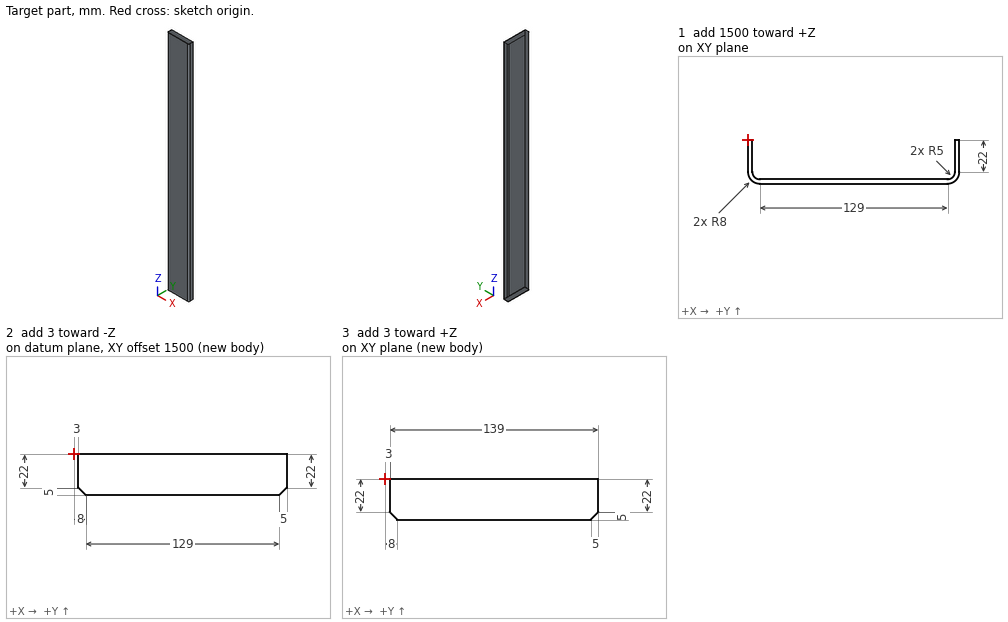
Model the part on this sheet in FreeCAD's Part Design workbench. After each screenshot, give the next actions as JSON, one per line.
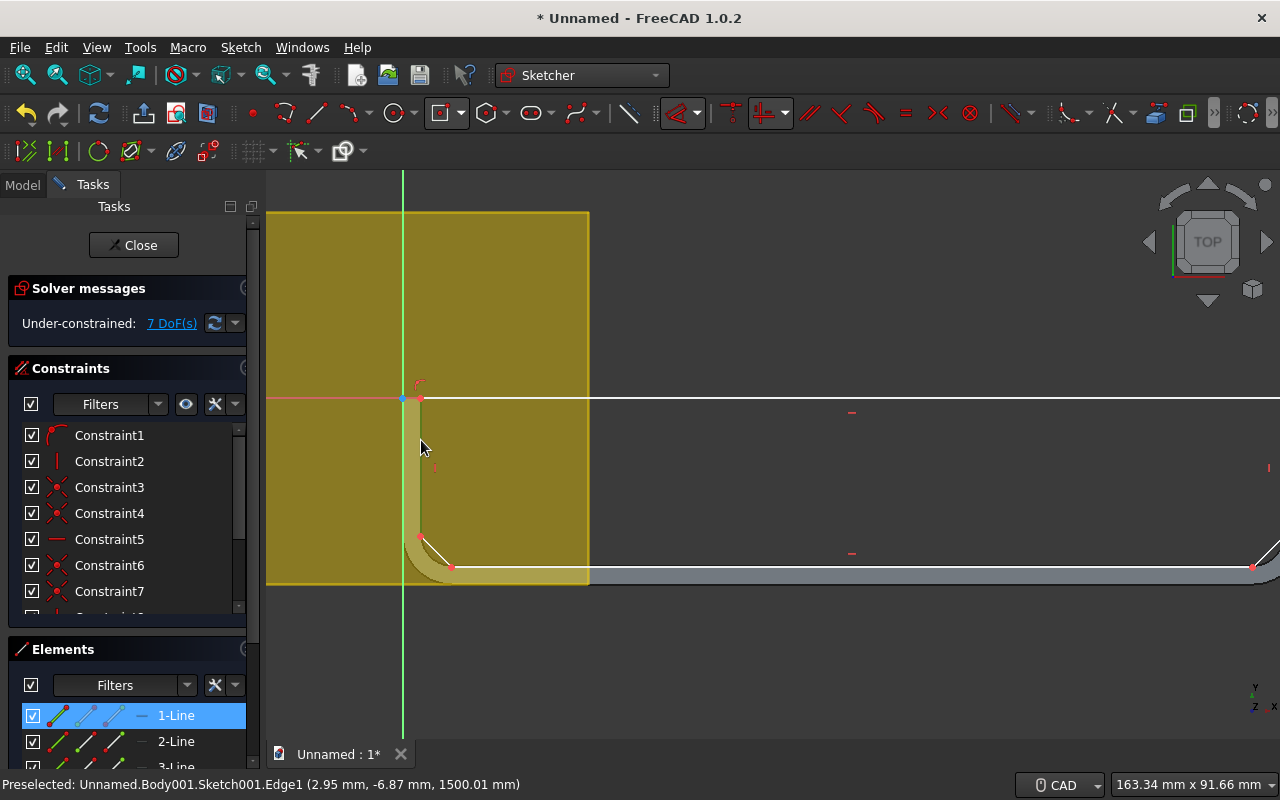
{"action": "key", "text": "i"}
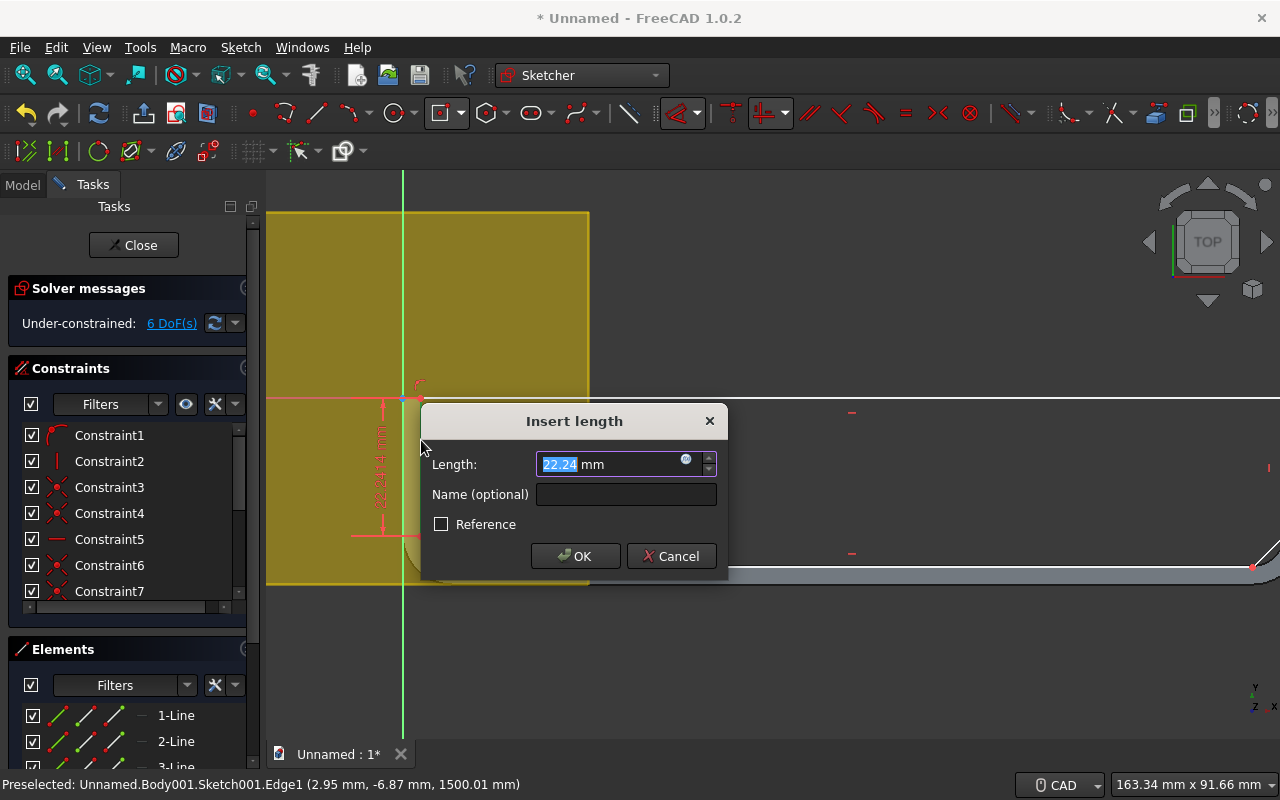
{"action": "type", "text": "22"}
{"action": "key", "text": "Return"}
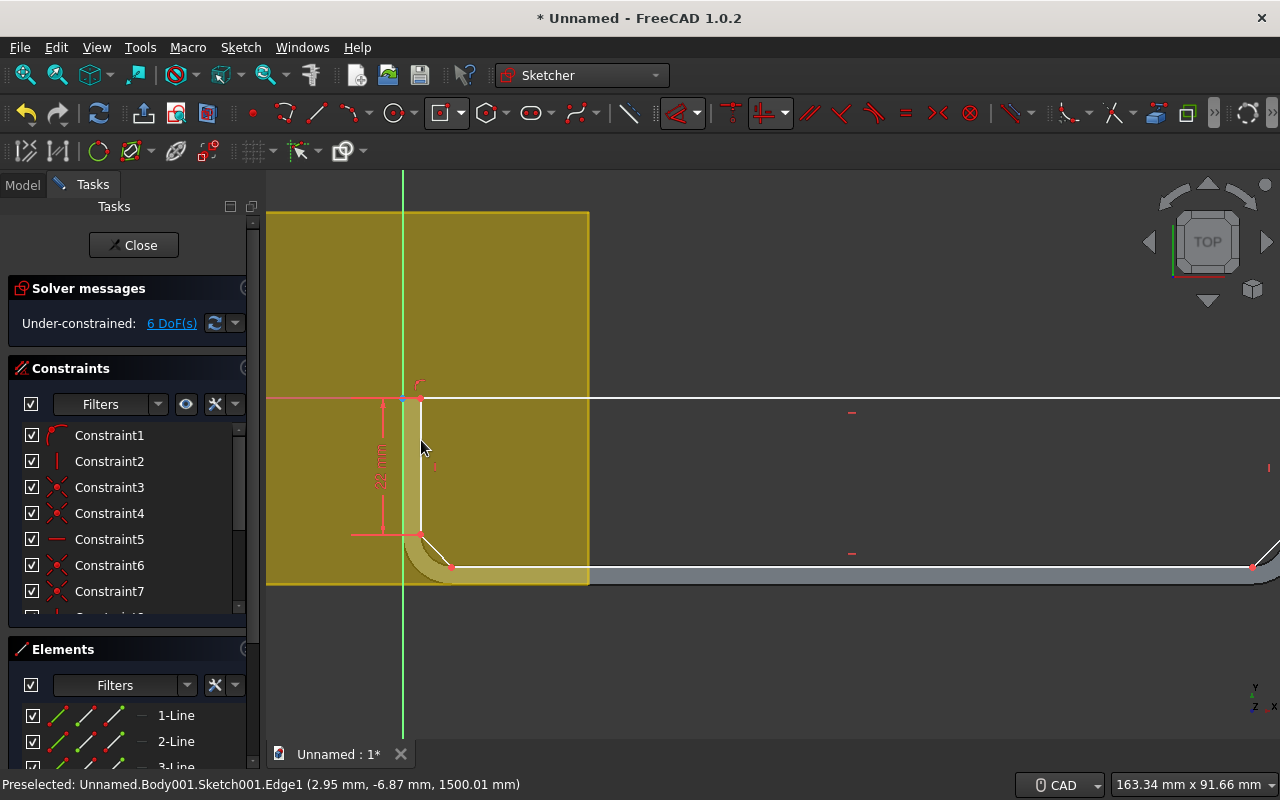
{"action": "scroll", "coordinate": [422, 398], "scroll_direction": "down", "scroll_amount": 2}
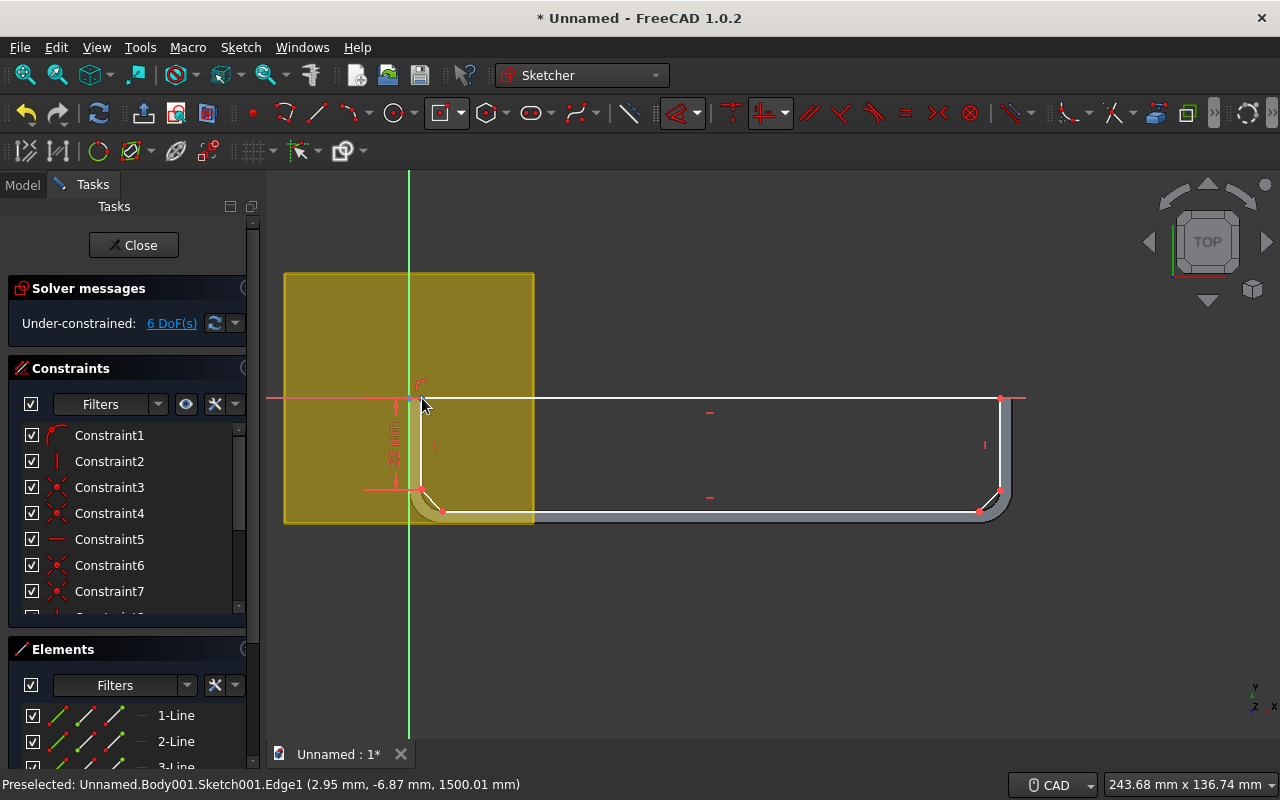
{"action": "left_click", "coordinate": [1000, 463]}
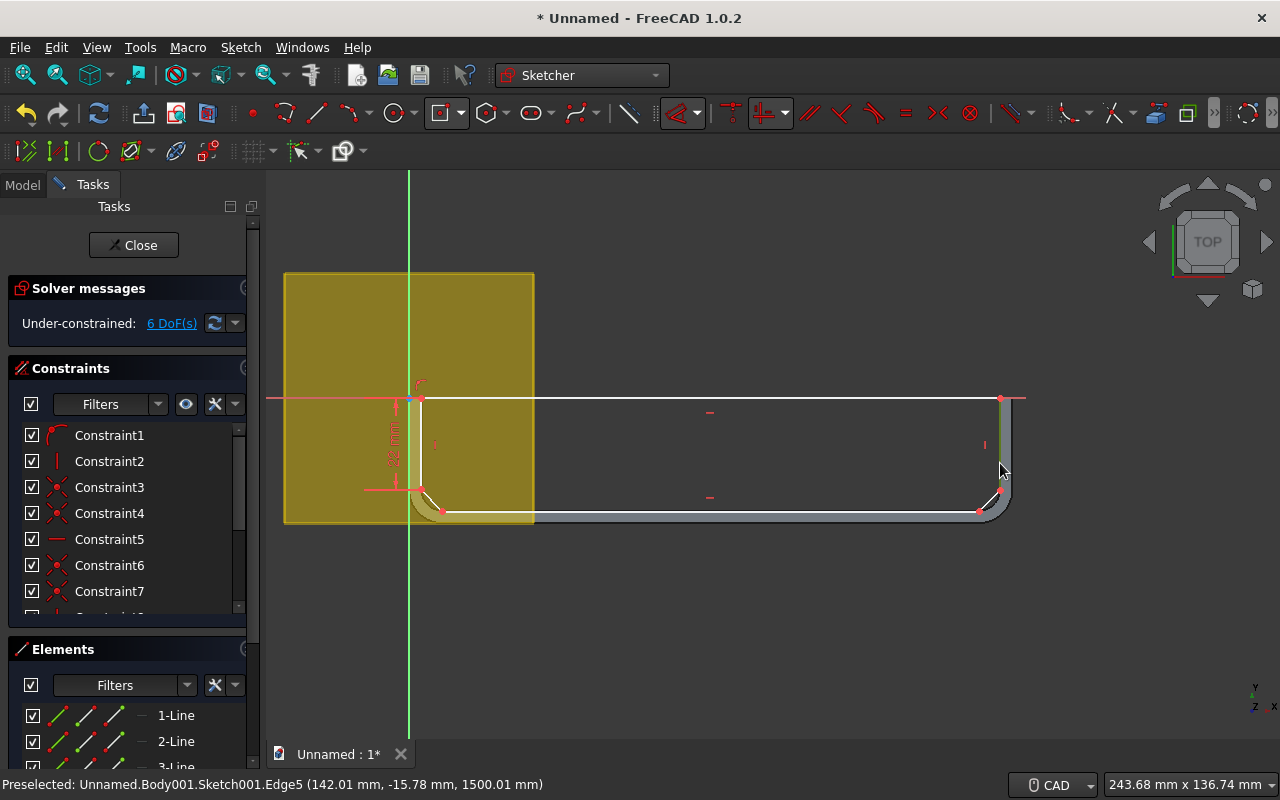
{"action": "left_click", "coordinate": [700, 114]}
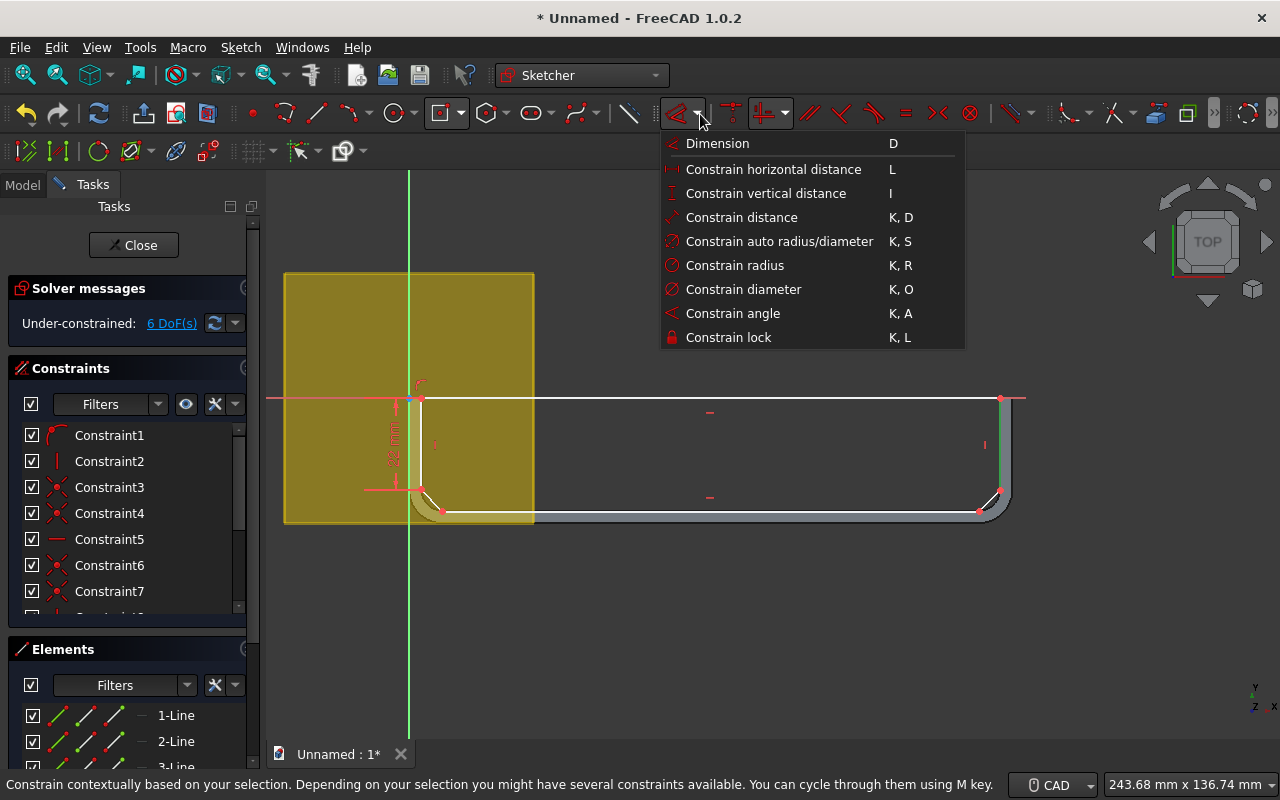
{"action": "left_click", "coordinate": [813, 193]}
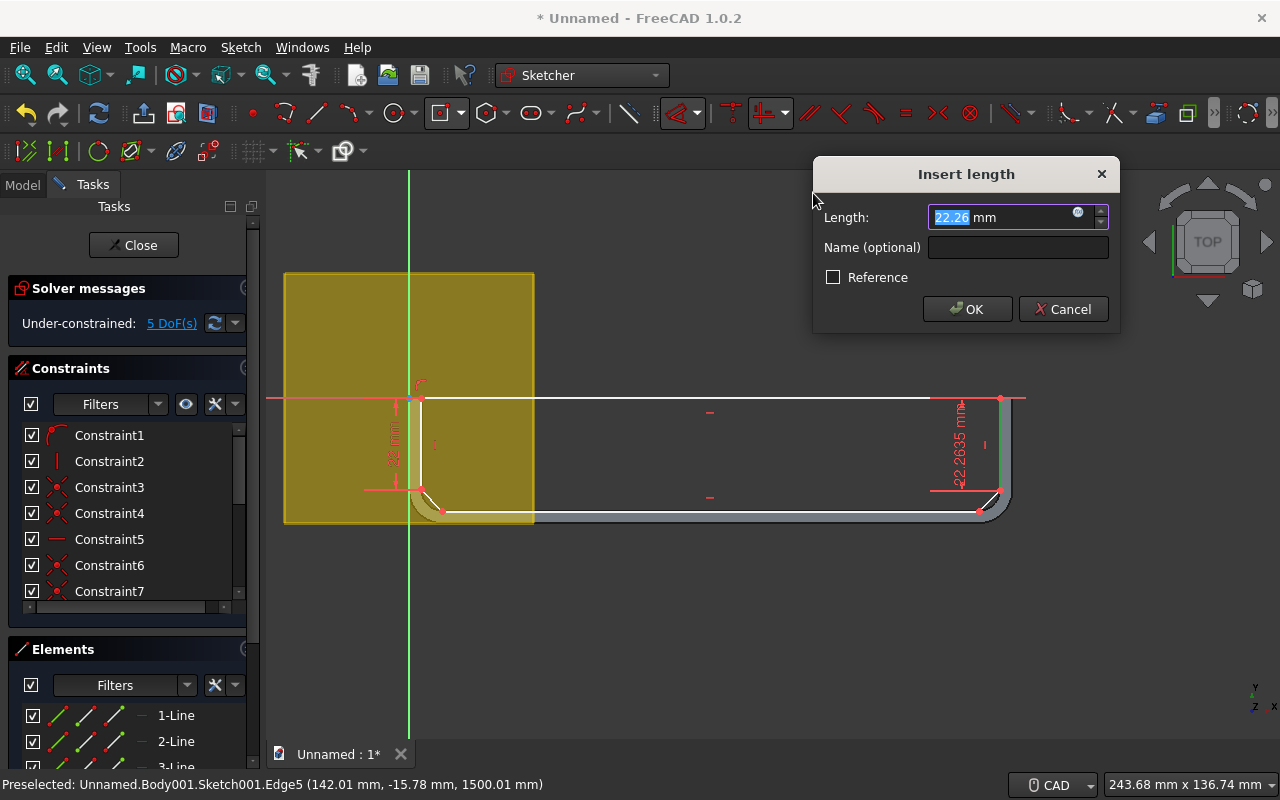
{"action": "type", "text": "22"}
{"action": "key", "text": "Return"}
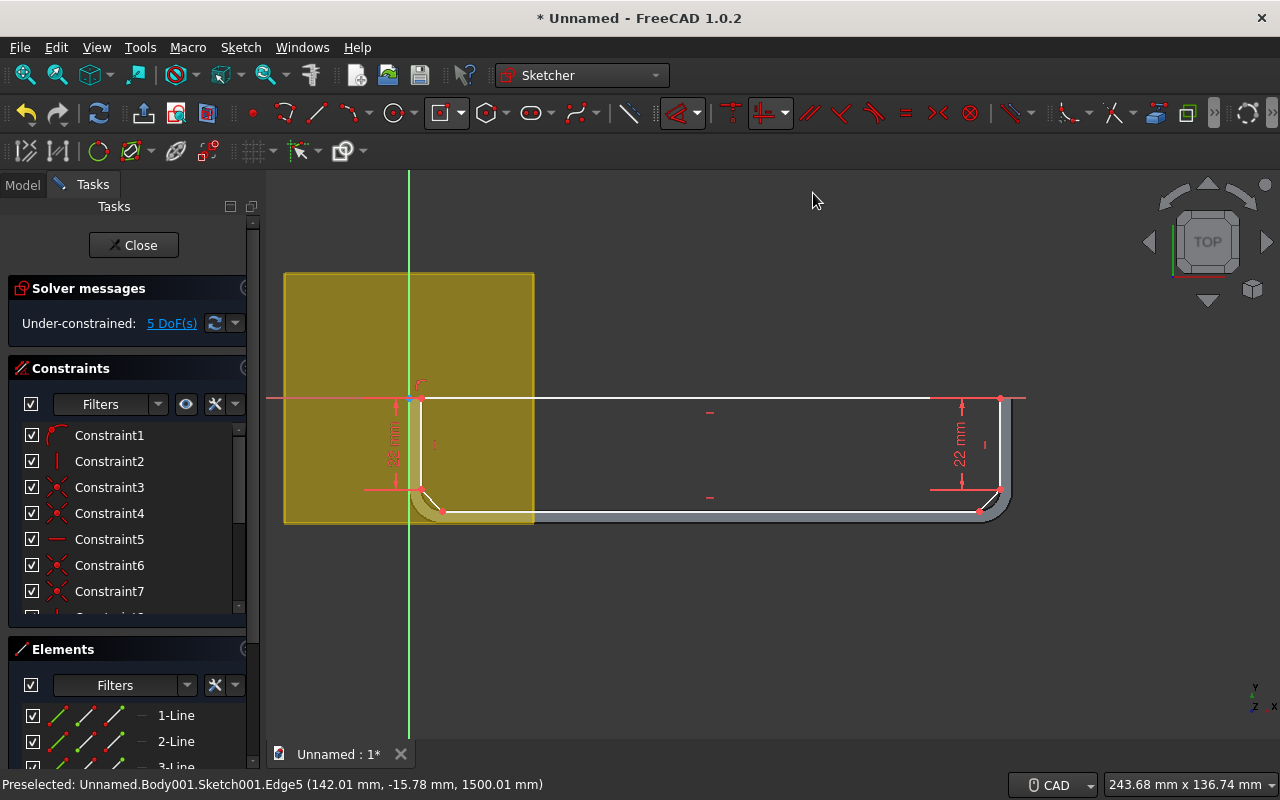
{"action": "scroll", "coordinate": [421, 398], "scroll_direction": "up", "scroll_amount": 6}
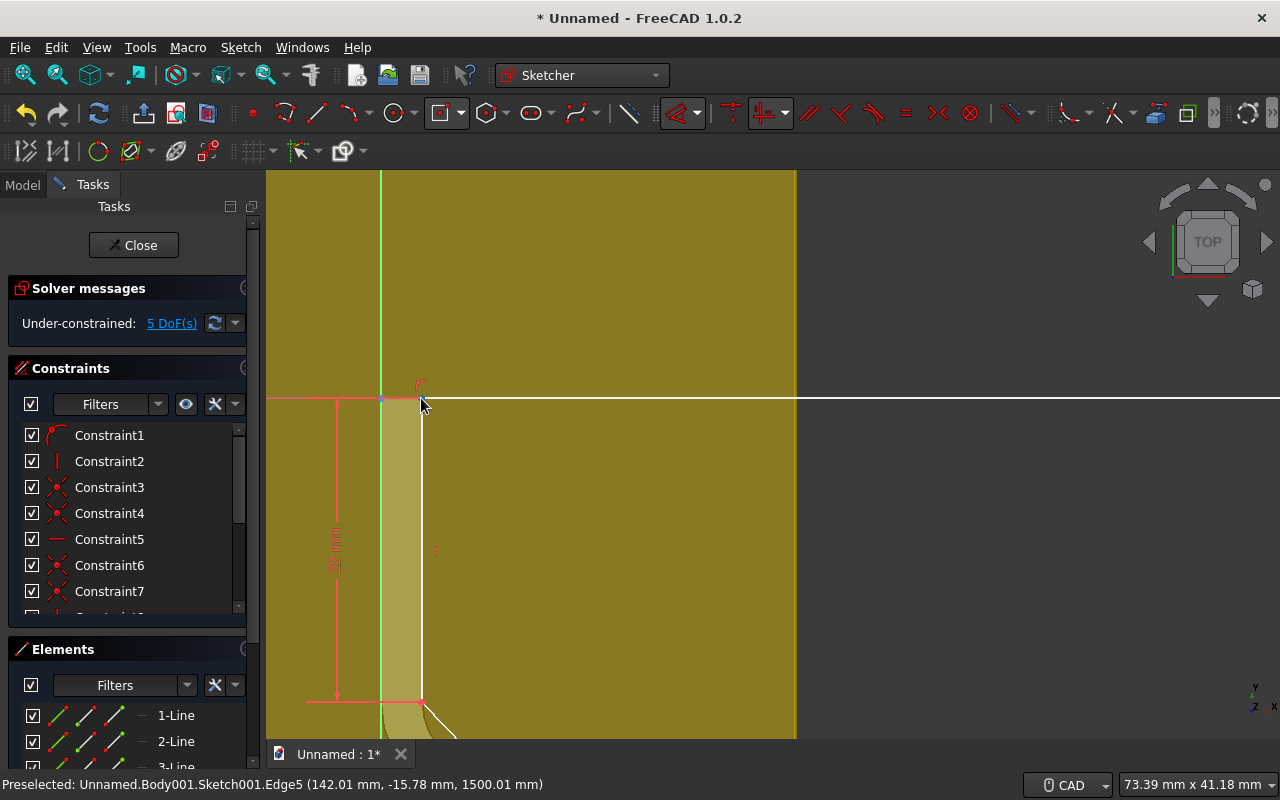
{"action": "left_click", "coordinate": [422, 398]}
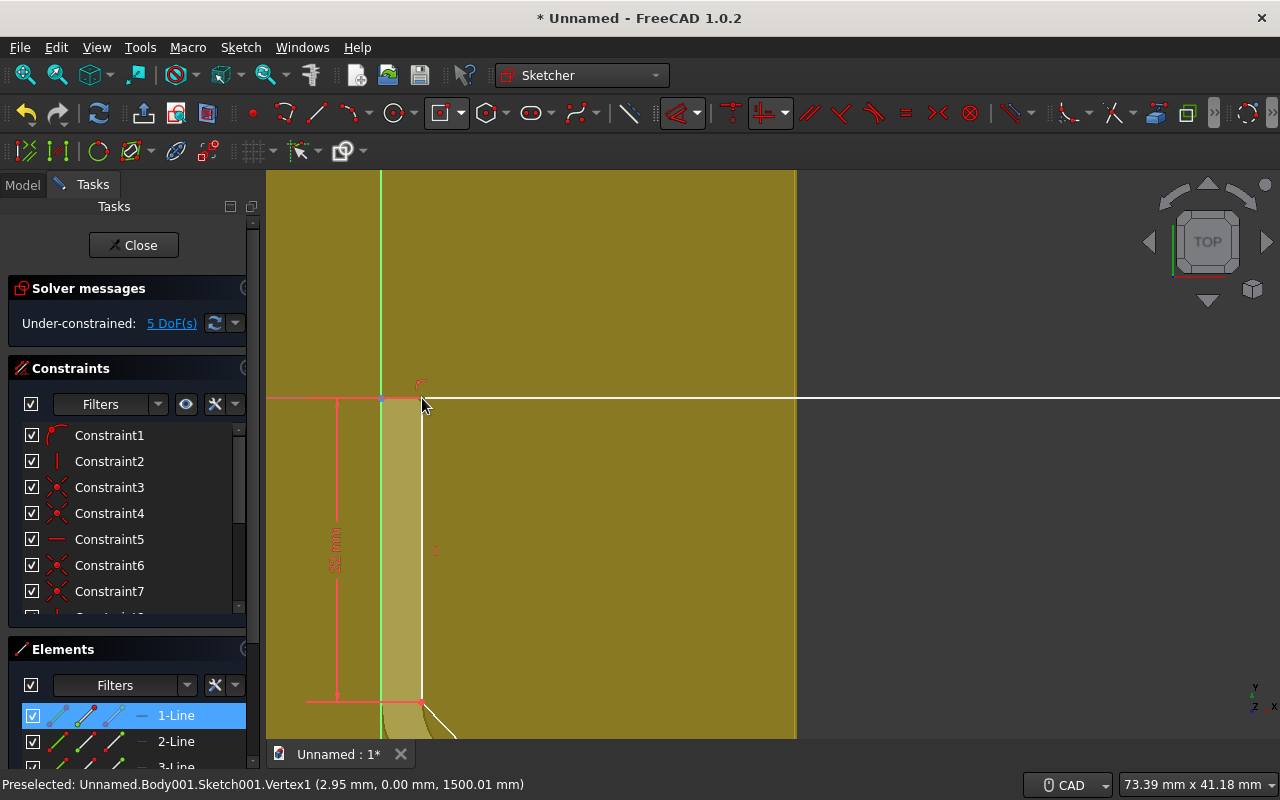
{"action": "key", "text": "l"}